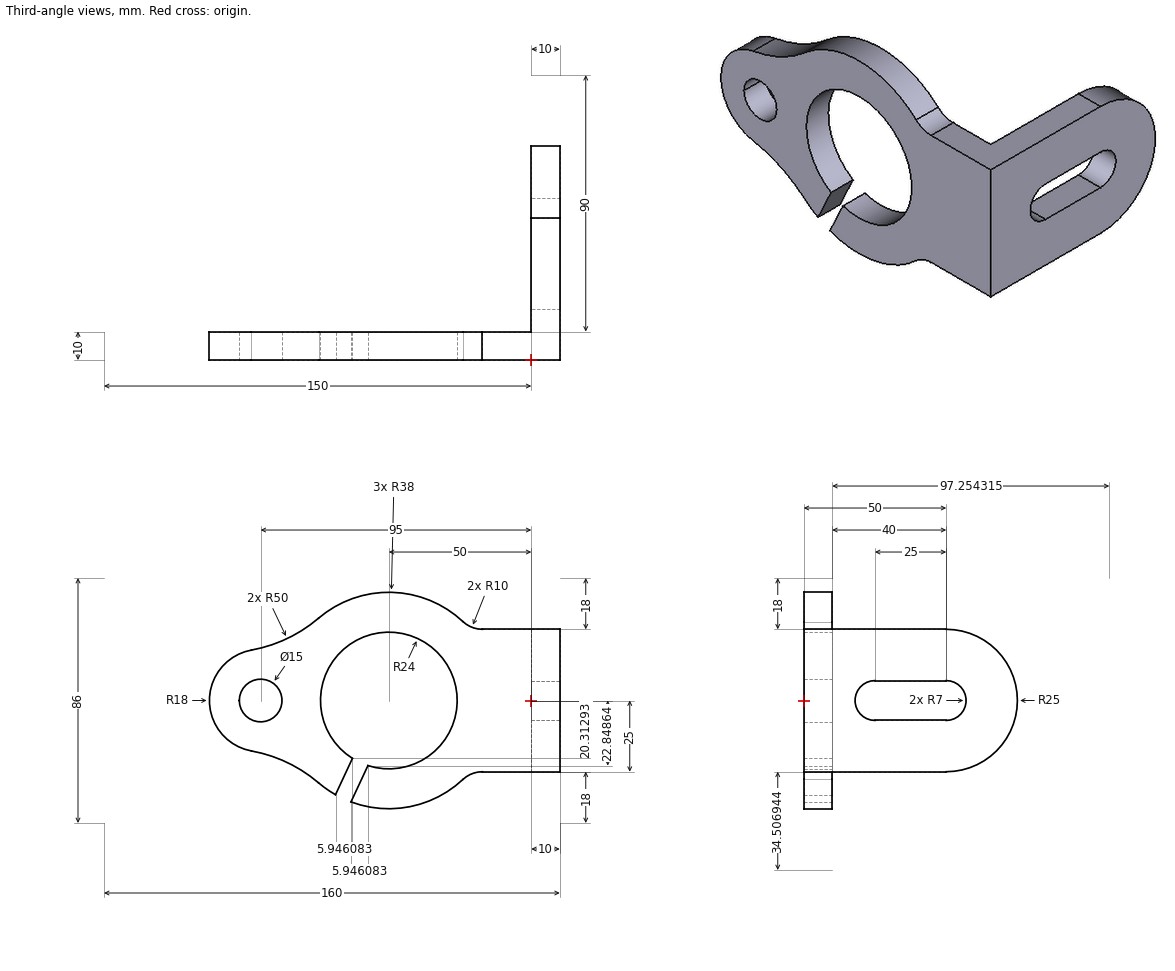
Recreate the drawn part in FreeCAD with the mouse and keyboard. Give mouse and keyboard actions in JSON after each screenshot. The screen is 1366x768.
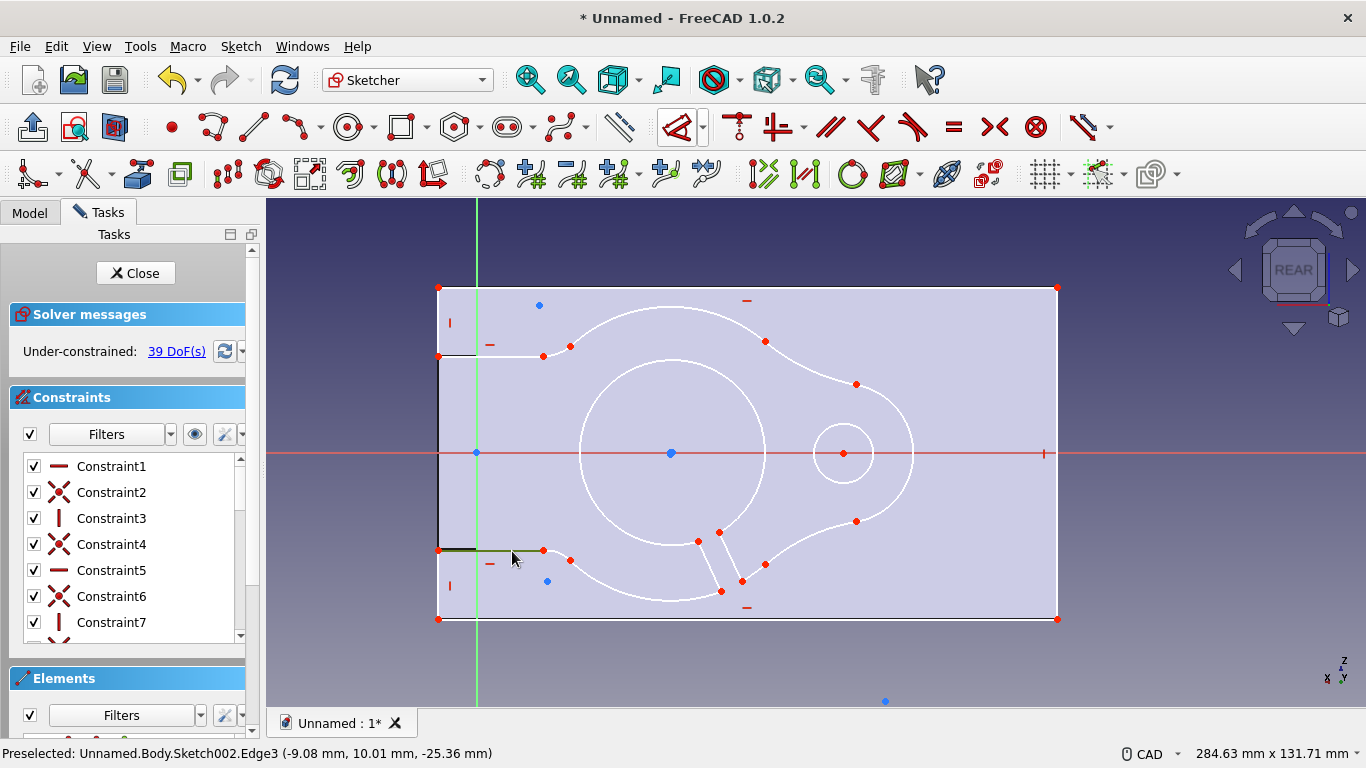
{"action": "left_click", "coordinate": [558, 552]}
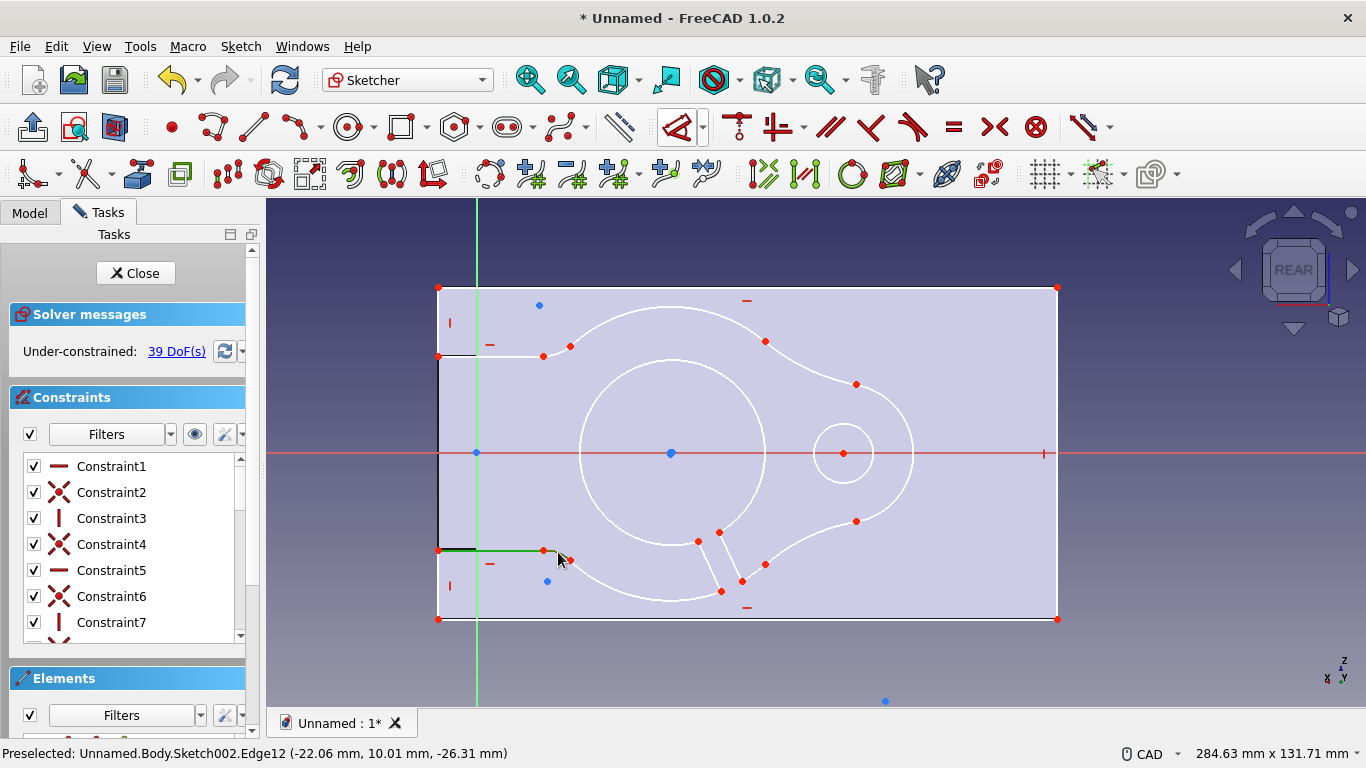
{"action": "key", "text": "t"}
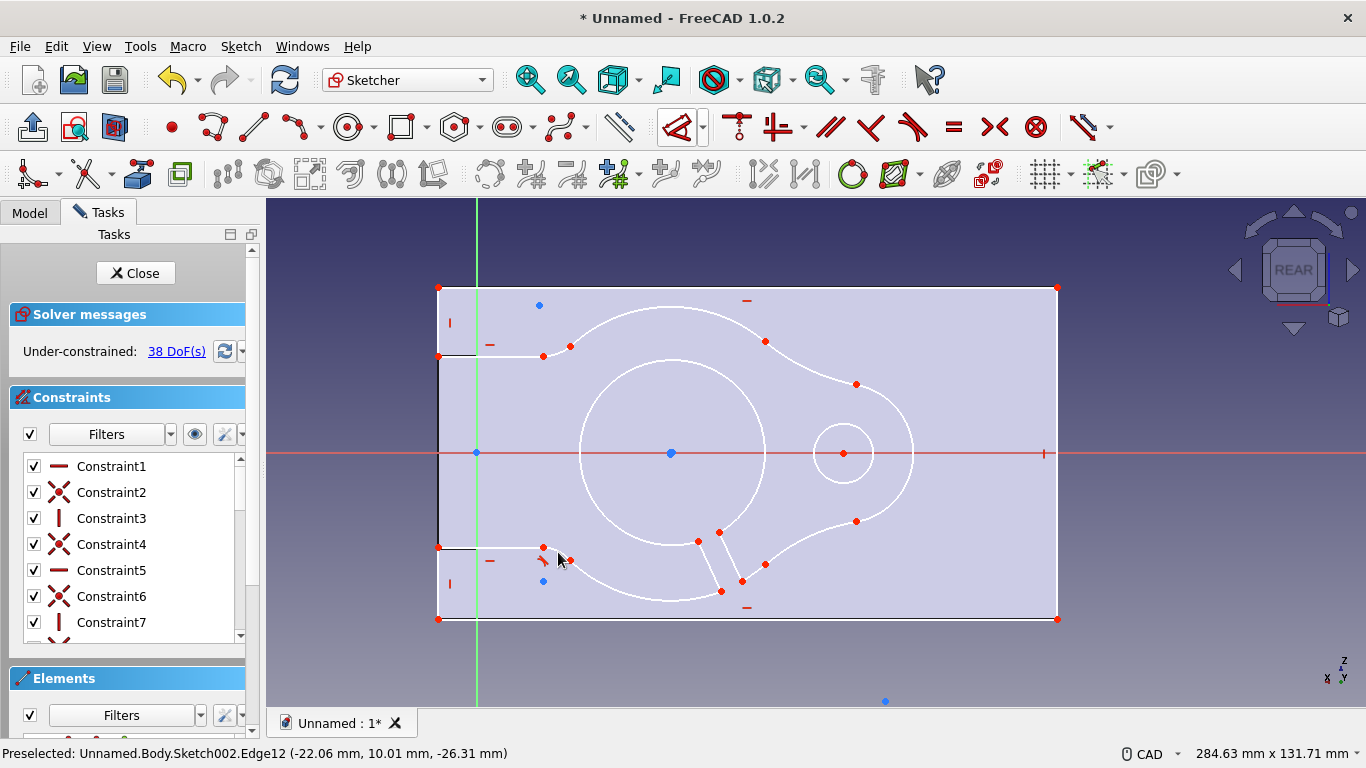
{"action": "left_click", "coordinate": [512, 357]}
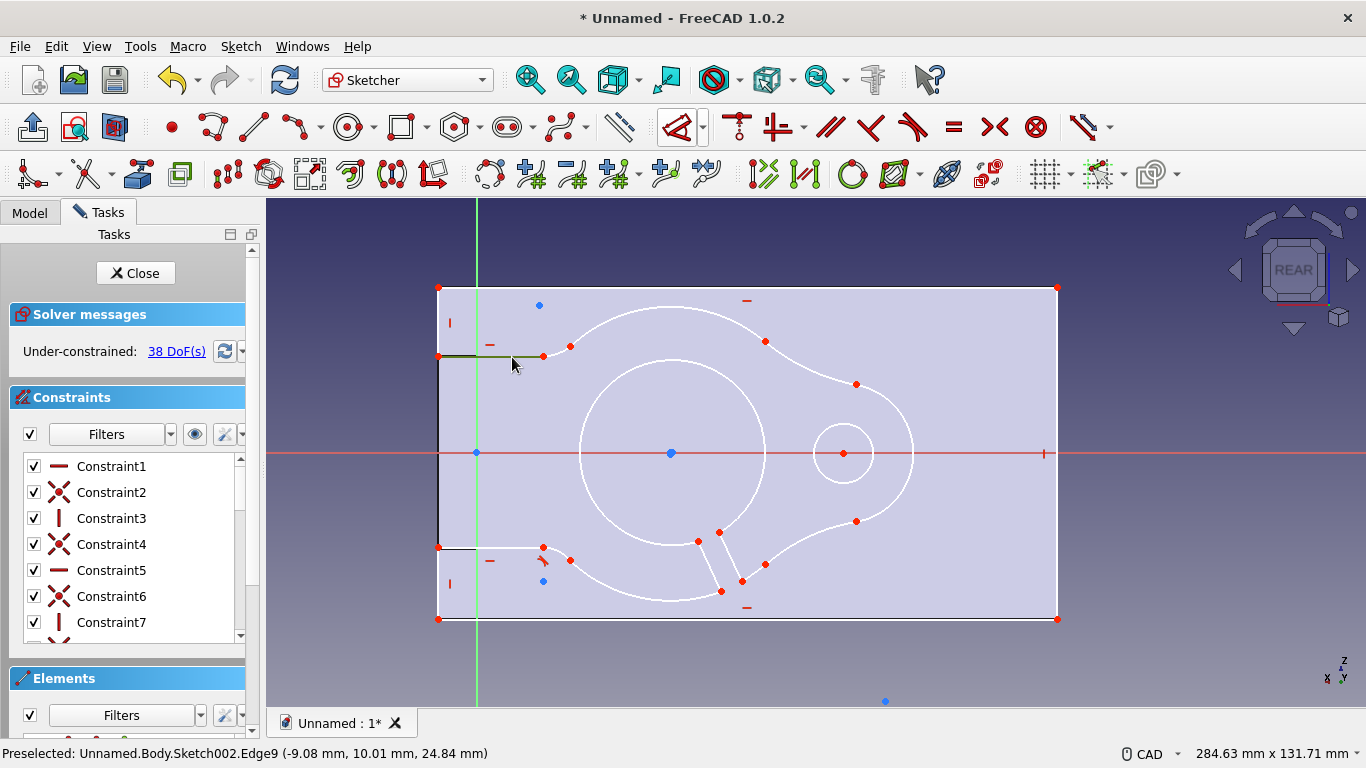
{"action": "left_click", "coordinate": [557, 354]}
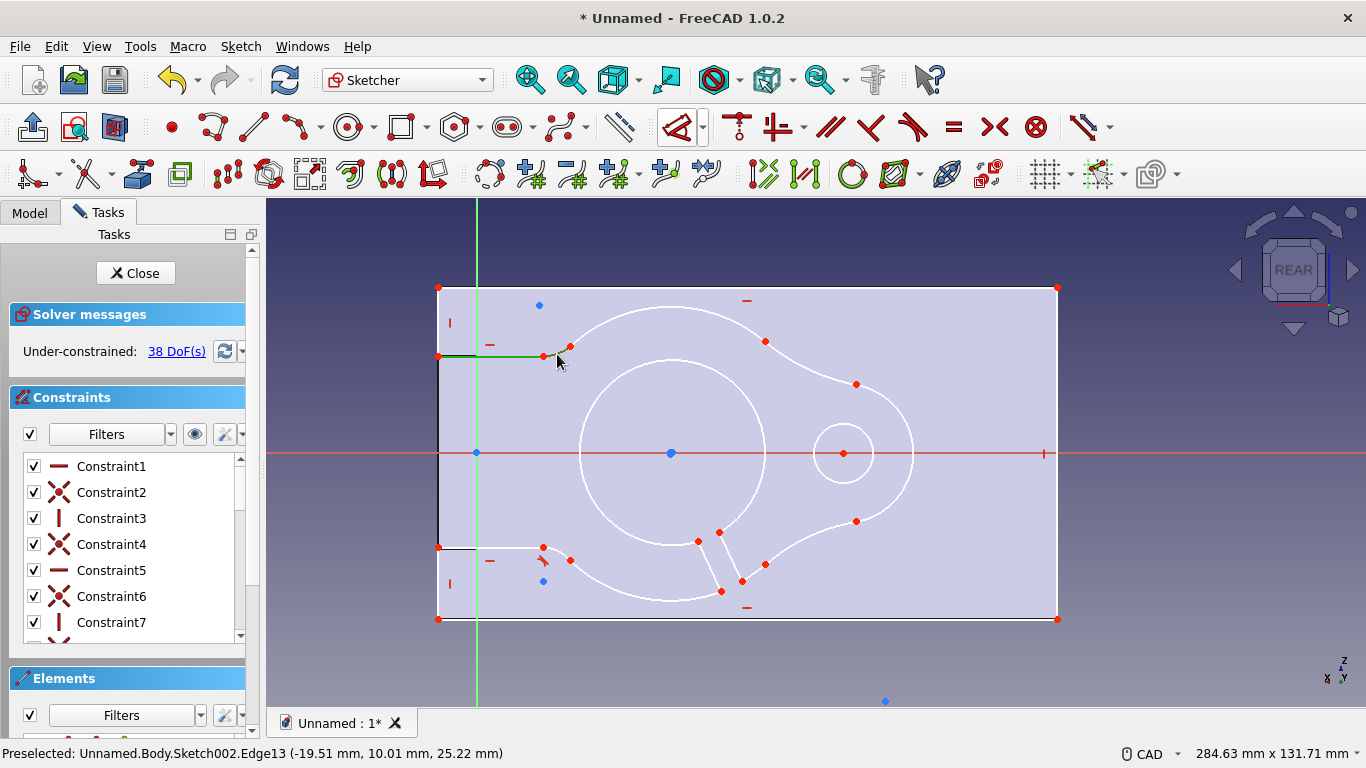
{"action": "key", "text": "t"}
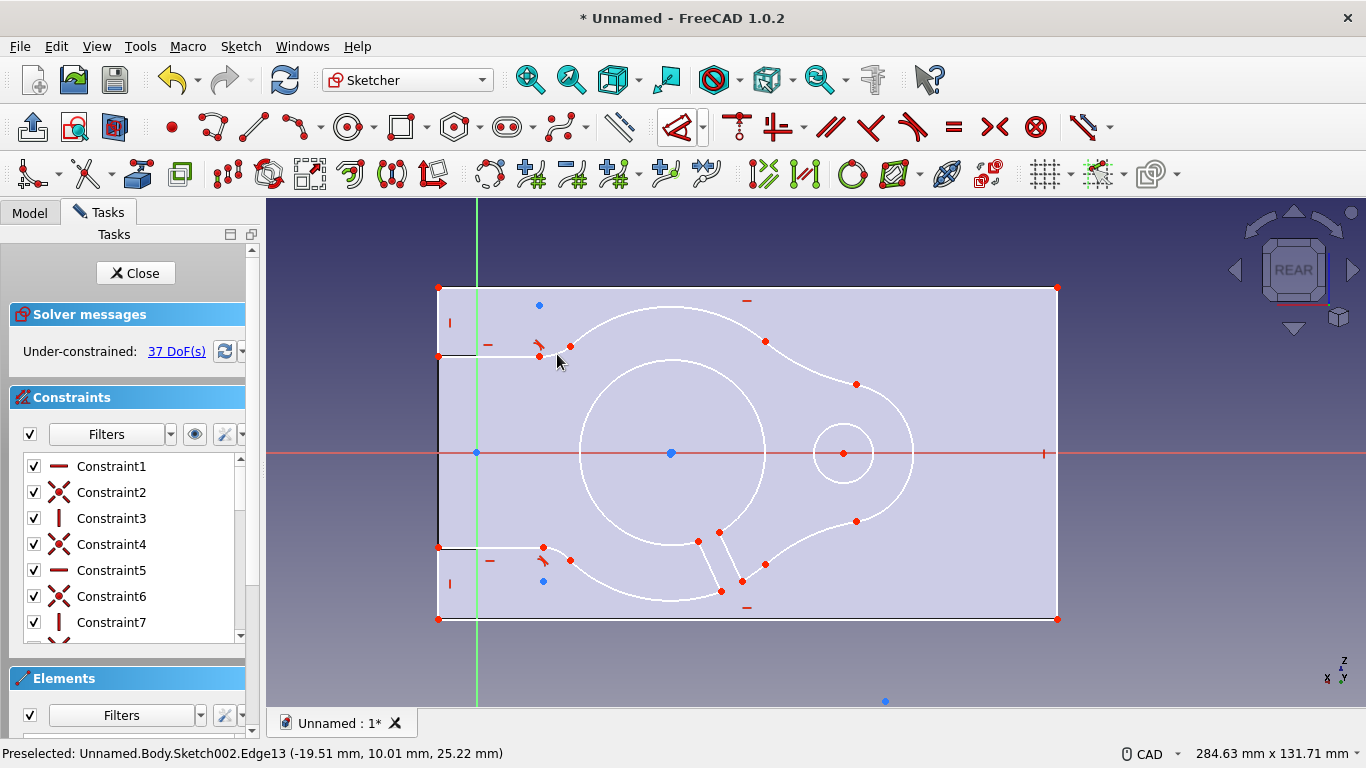
{"action": "left_click", "coordinate": [610, 588]}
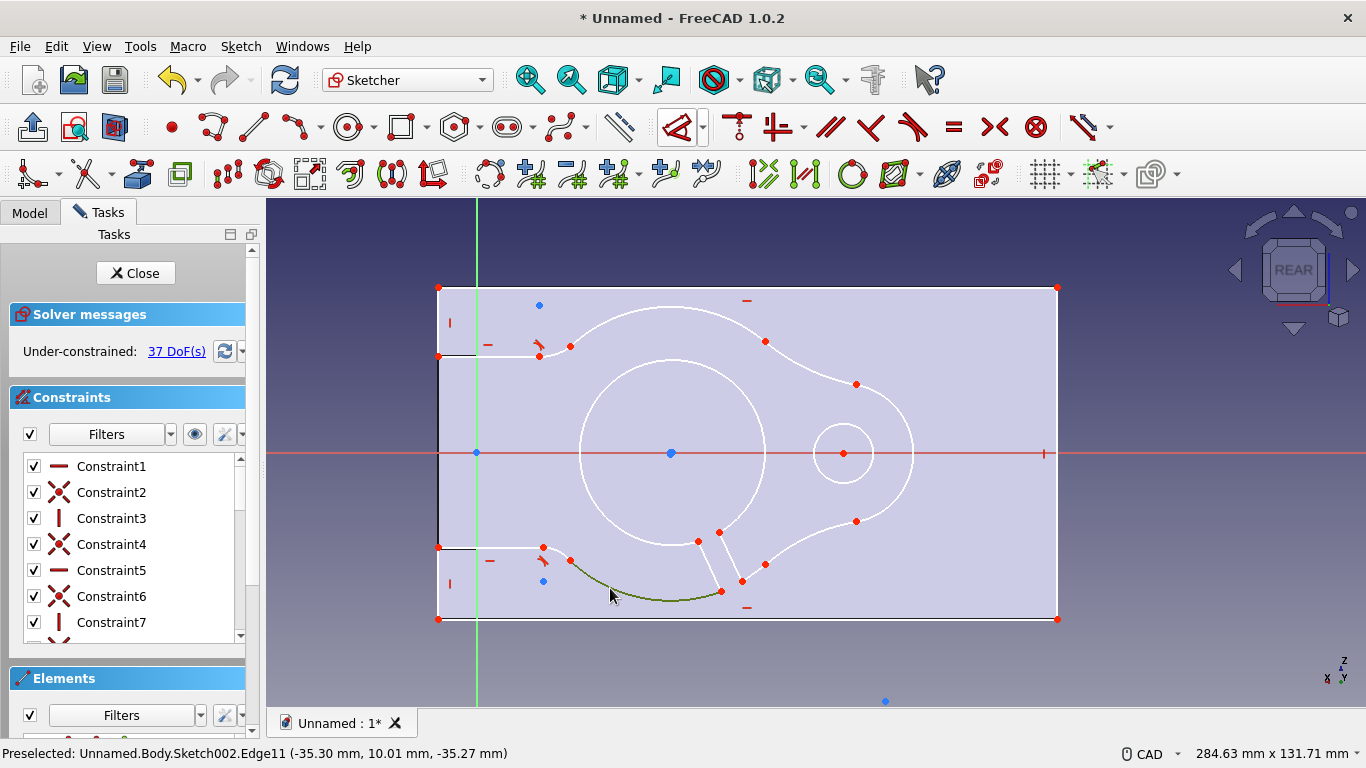
{"action": "scroll", "coordinate": [563, 554], "scroll_direction": "up", "scroll_amount": 2}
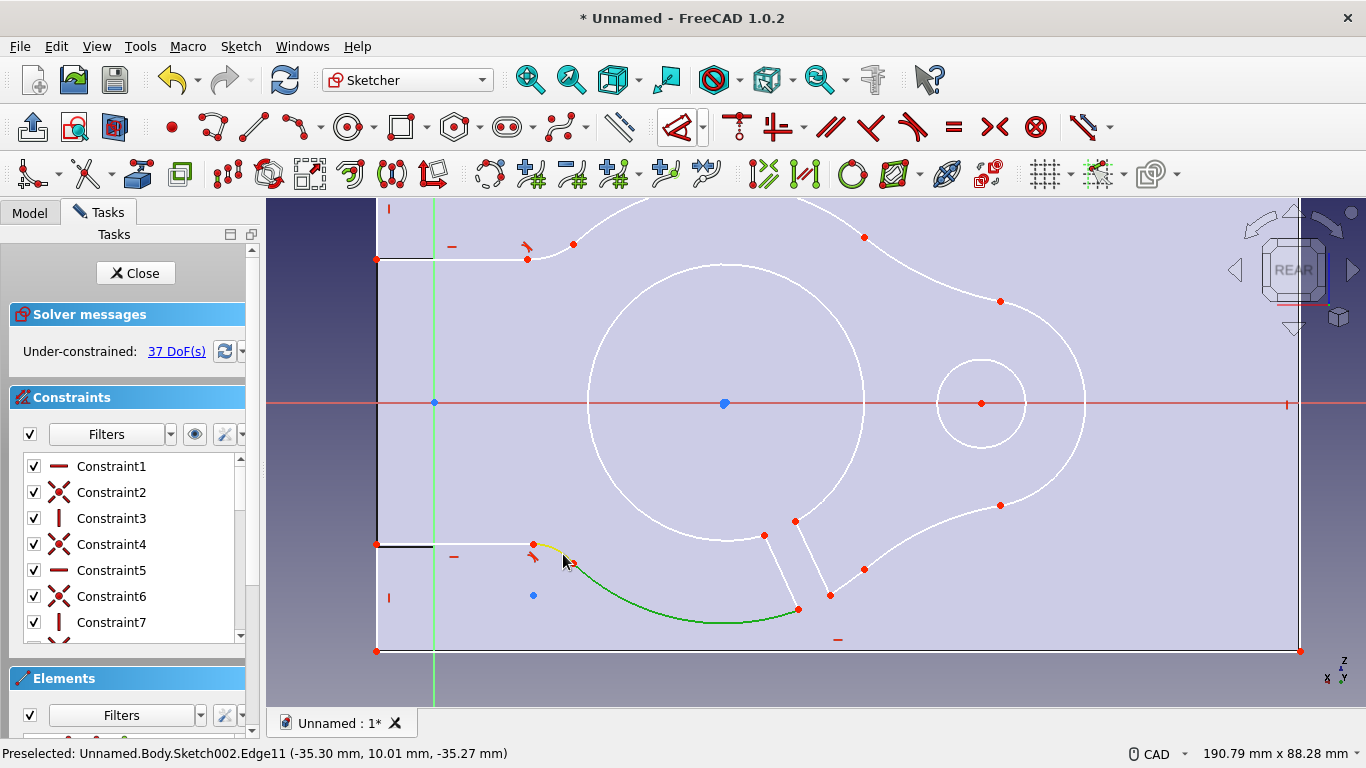
{"action": "left_click", "coordinate": [564, 554]}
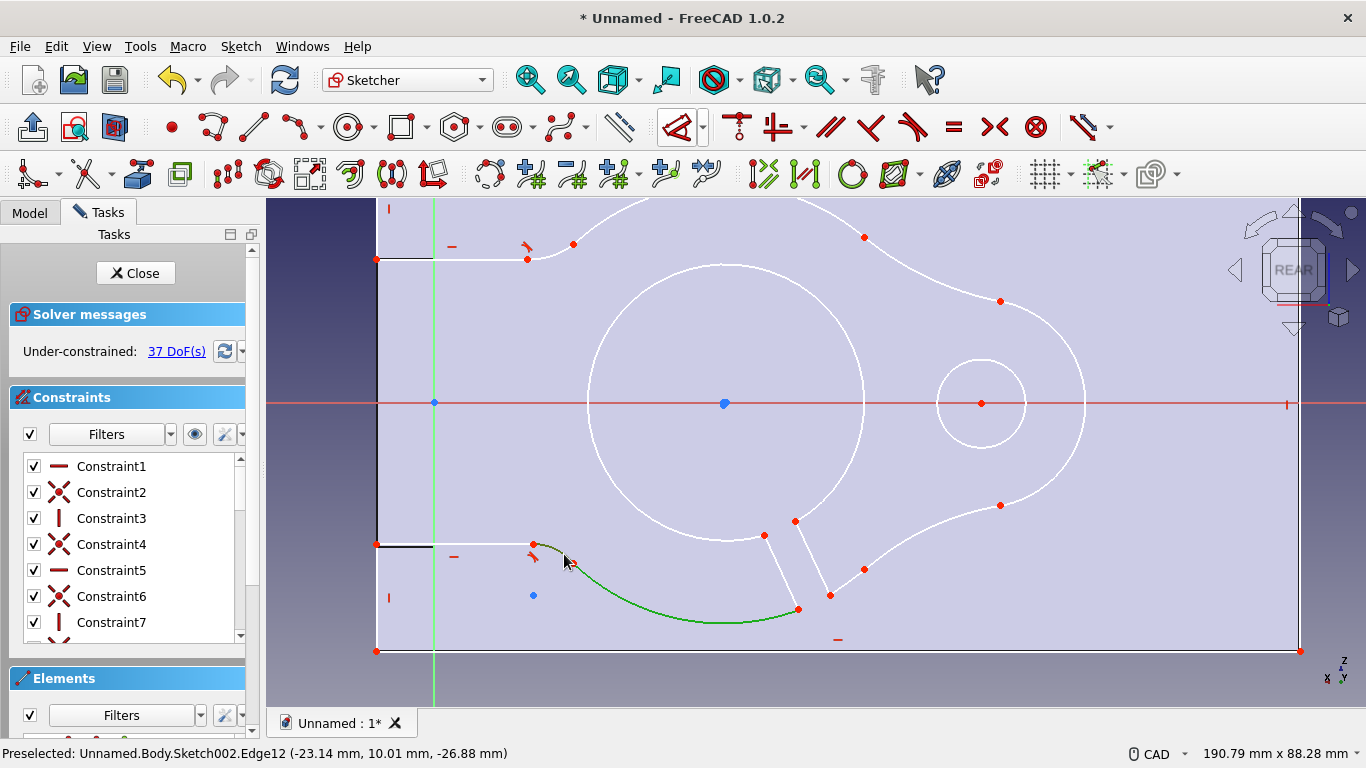
{"action": "key", "text": "t"}